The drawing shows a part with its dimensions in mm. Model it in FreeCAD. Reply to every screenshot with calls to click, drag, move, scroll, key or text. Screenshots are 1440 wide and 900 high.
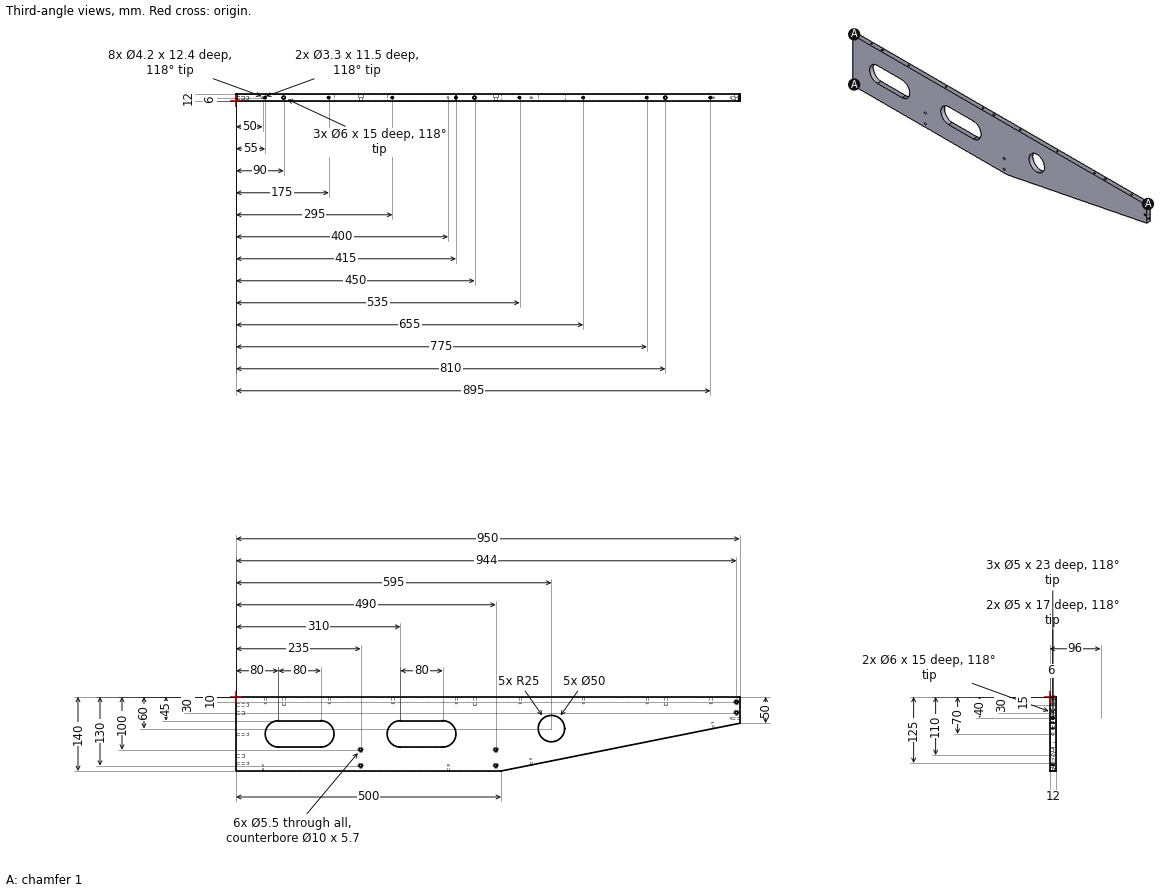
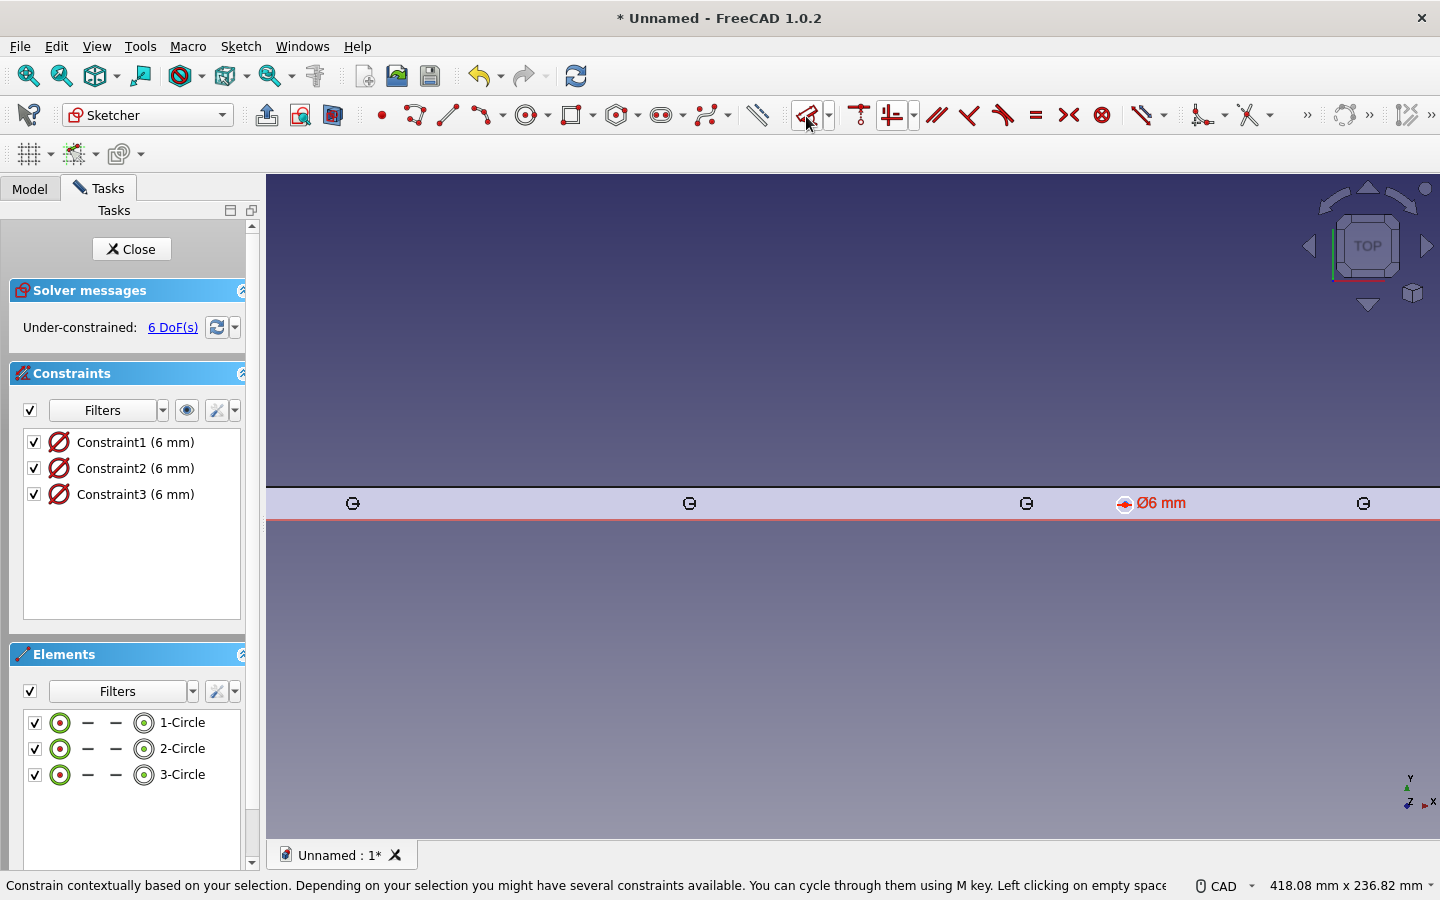
scroll(1126, 506, down, 6)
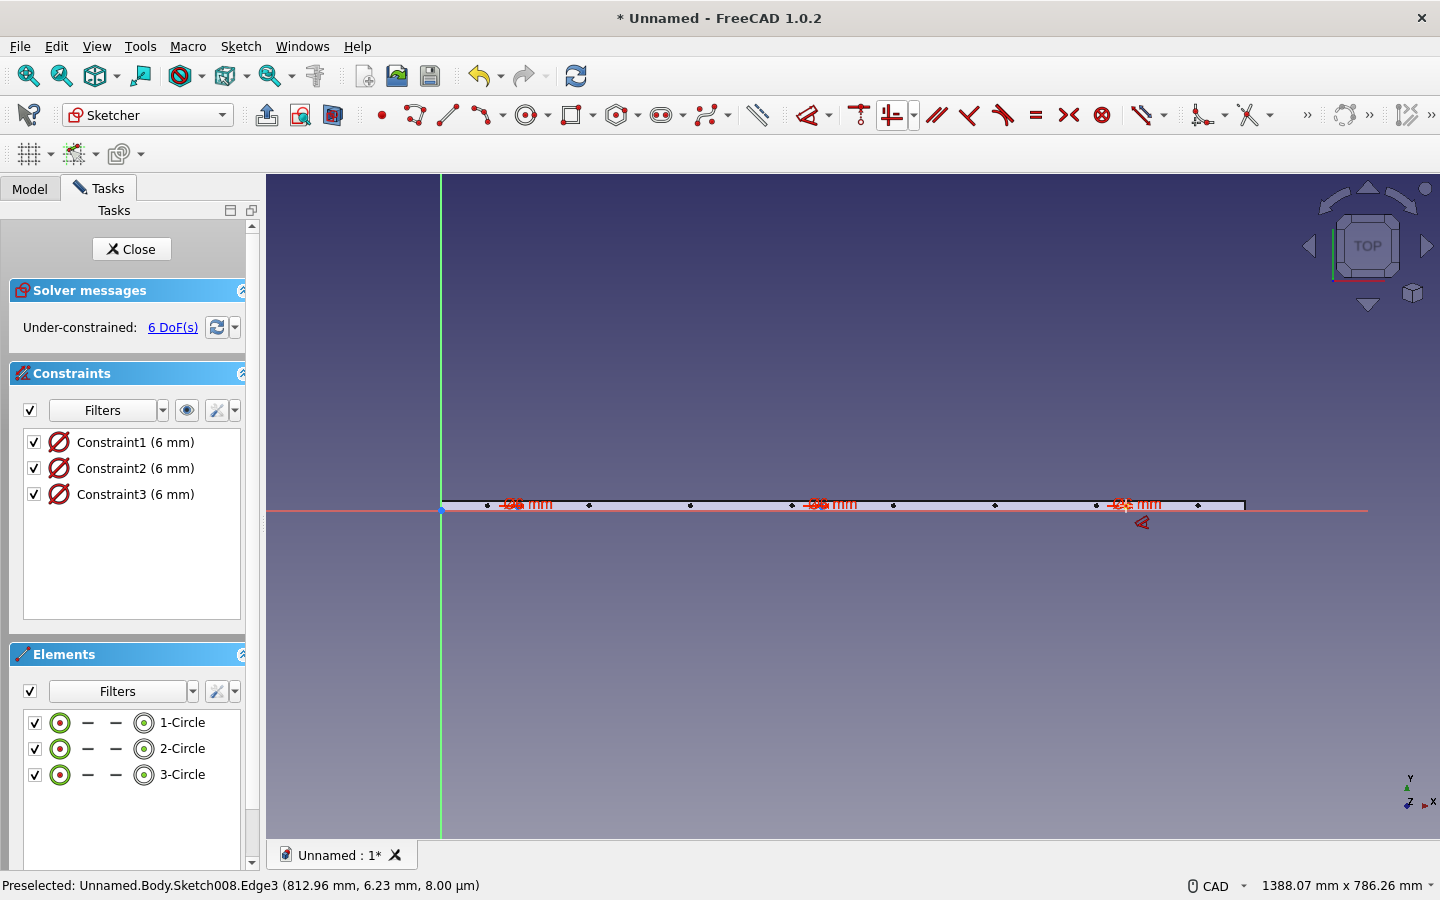
scroll(517, 506, up, 11)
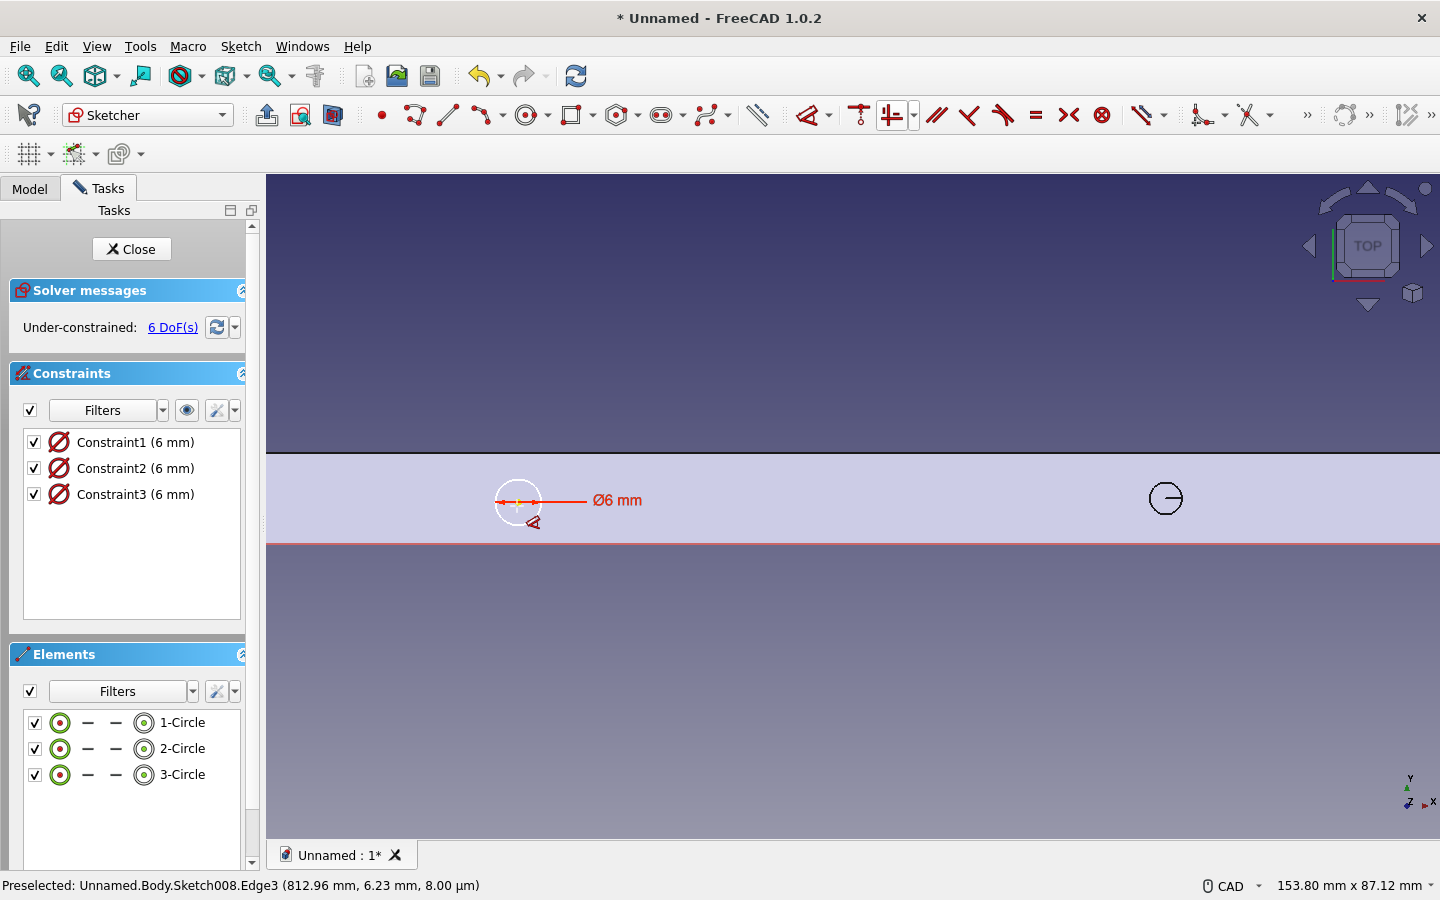
click(518, 502)
click(552, 523)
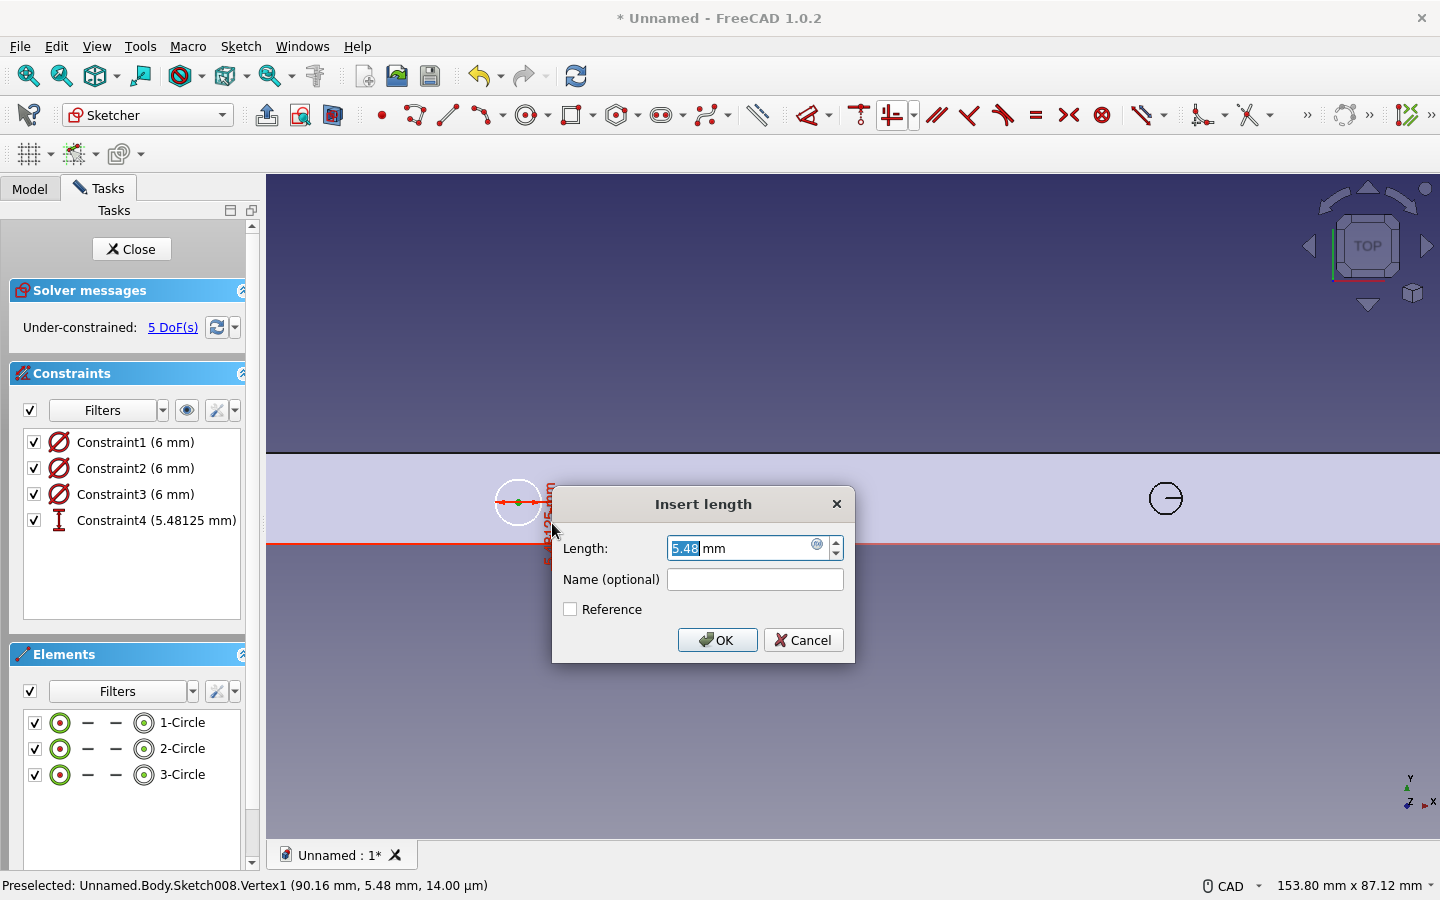
text(6)
key(Return)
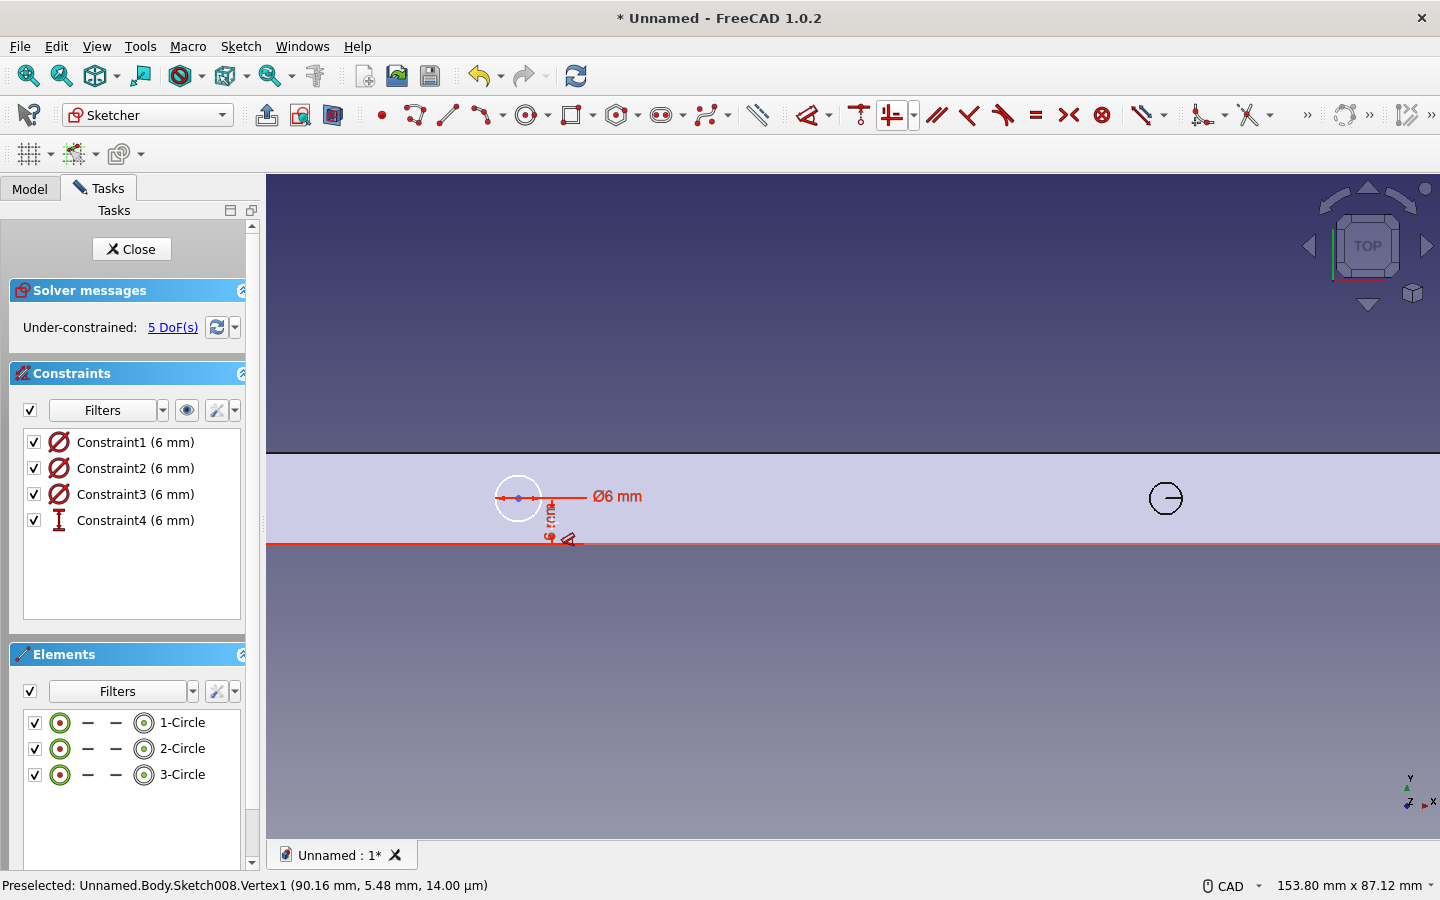
scroll(517, 506, down, 11)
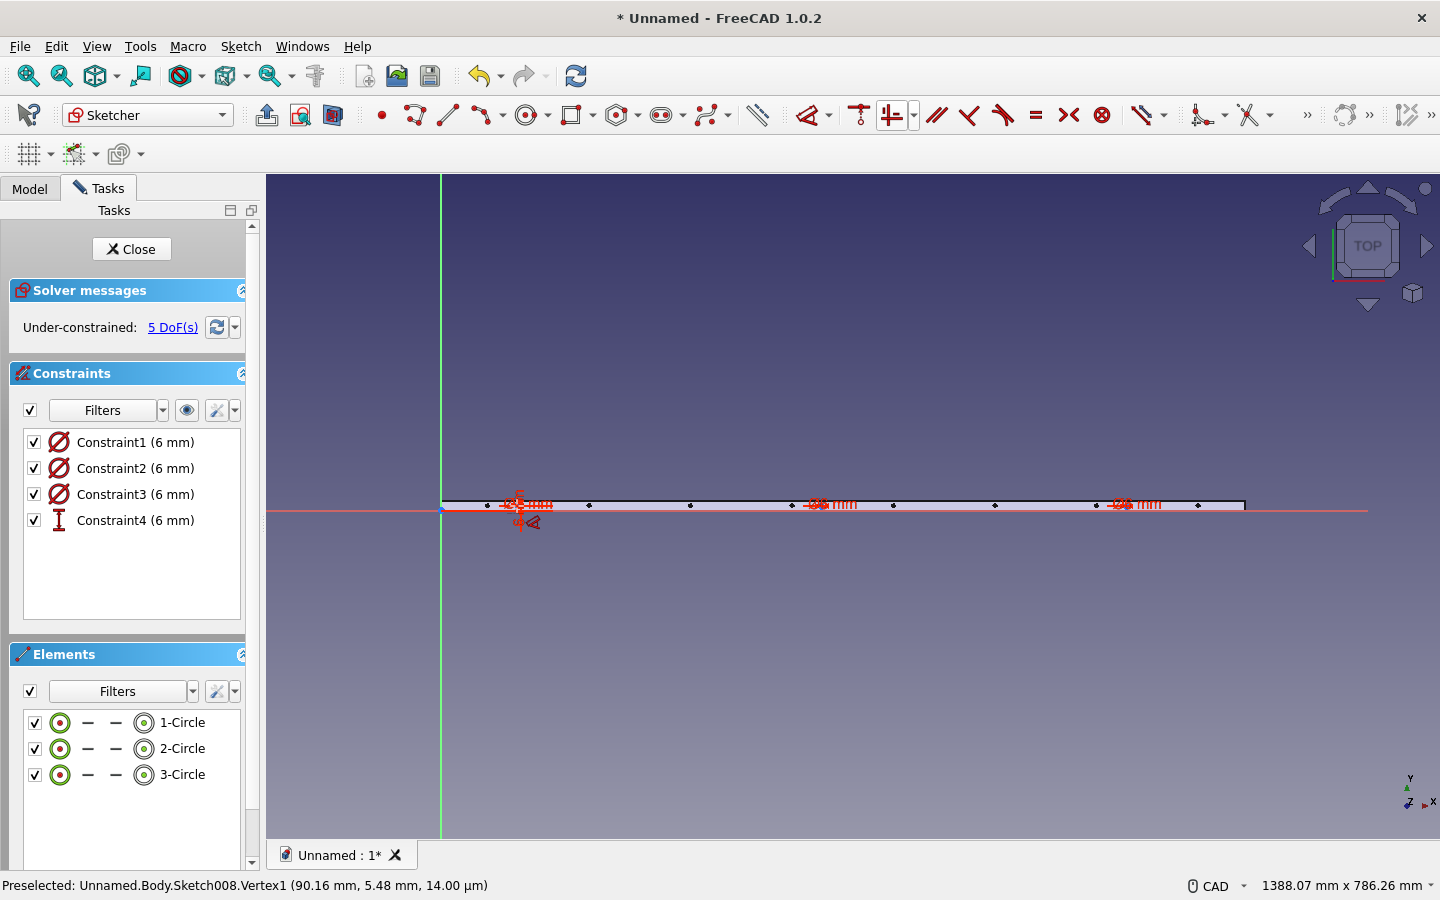
scroll(822, 506, up, 11)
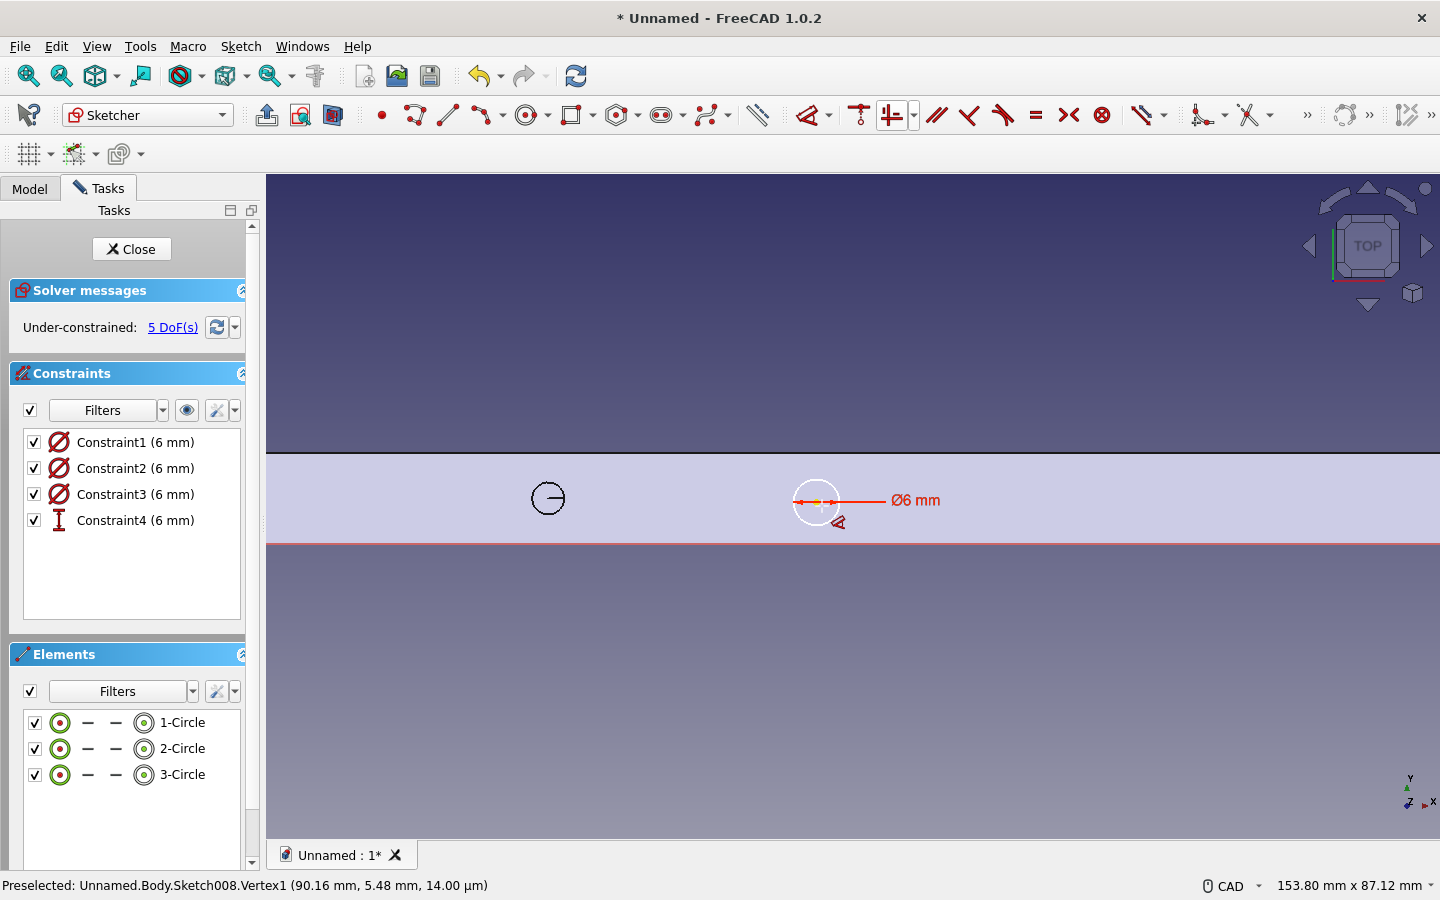
click(817, 502)
click(851, 523)